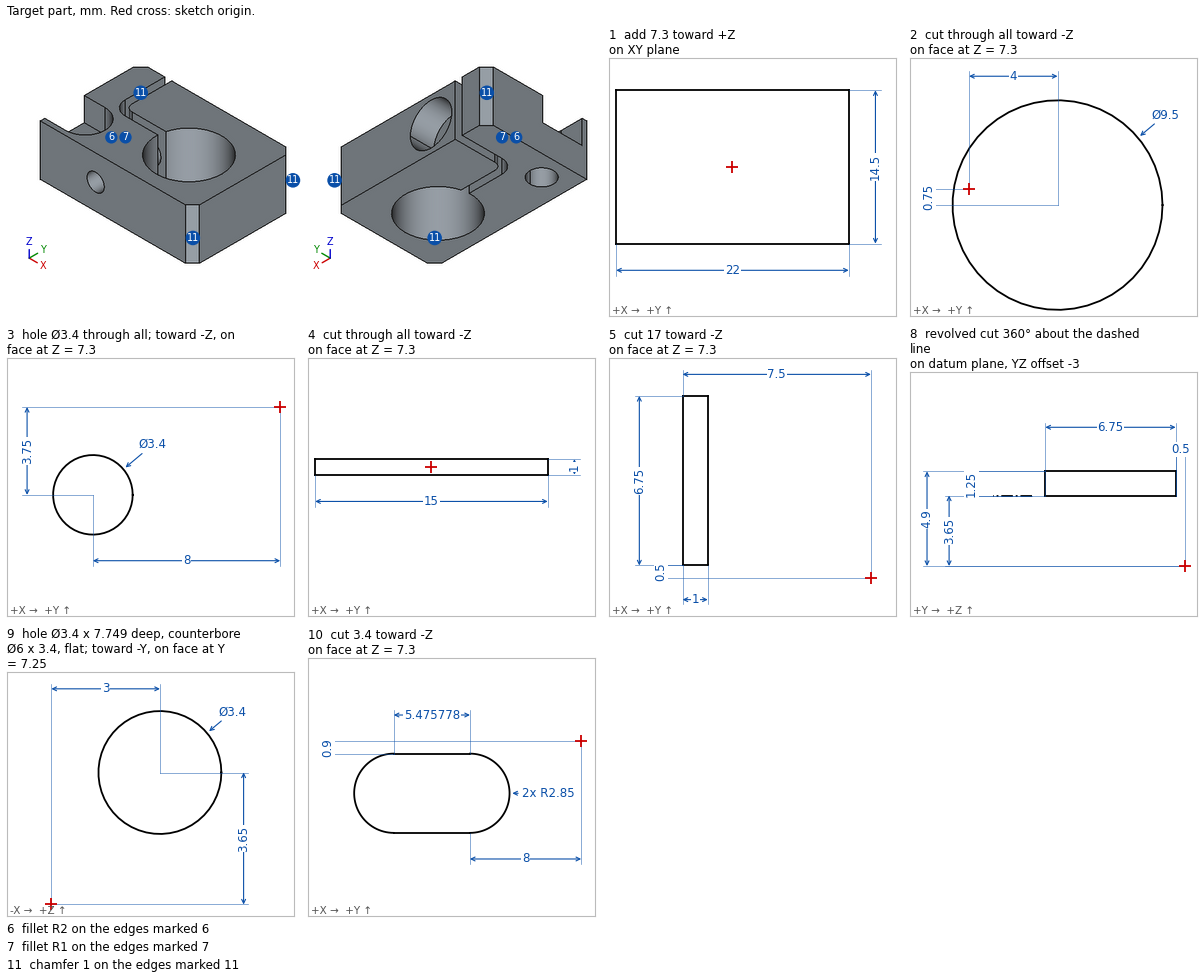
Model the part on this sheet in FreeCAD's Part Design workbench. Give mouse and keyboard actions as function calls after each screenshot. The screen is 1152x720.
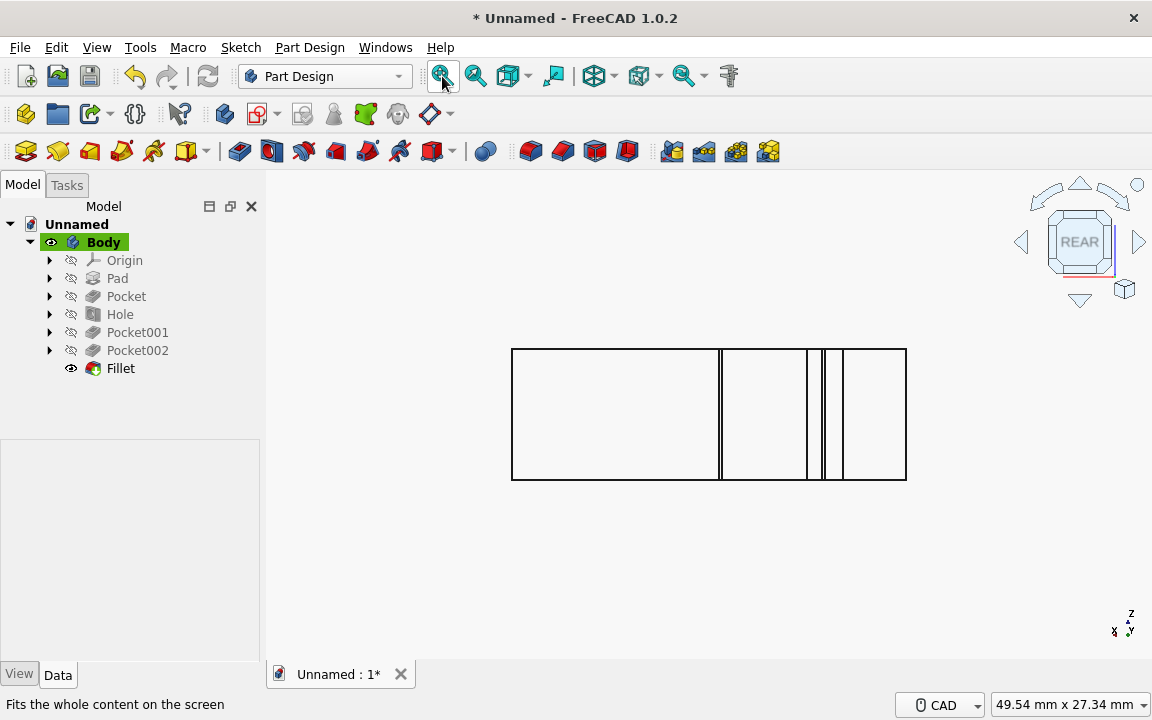
key(6)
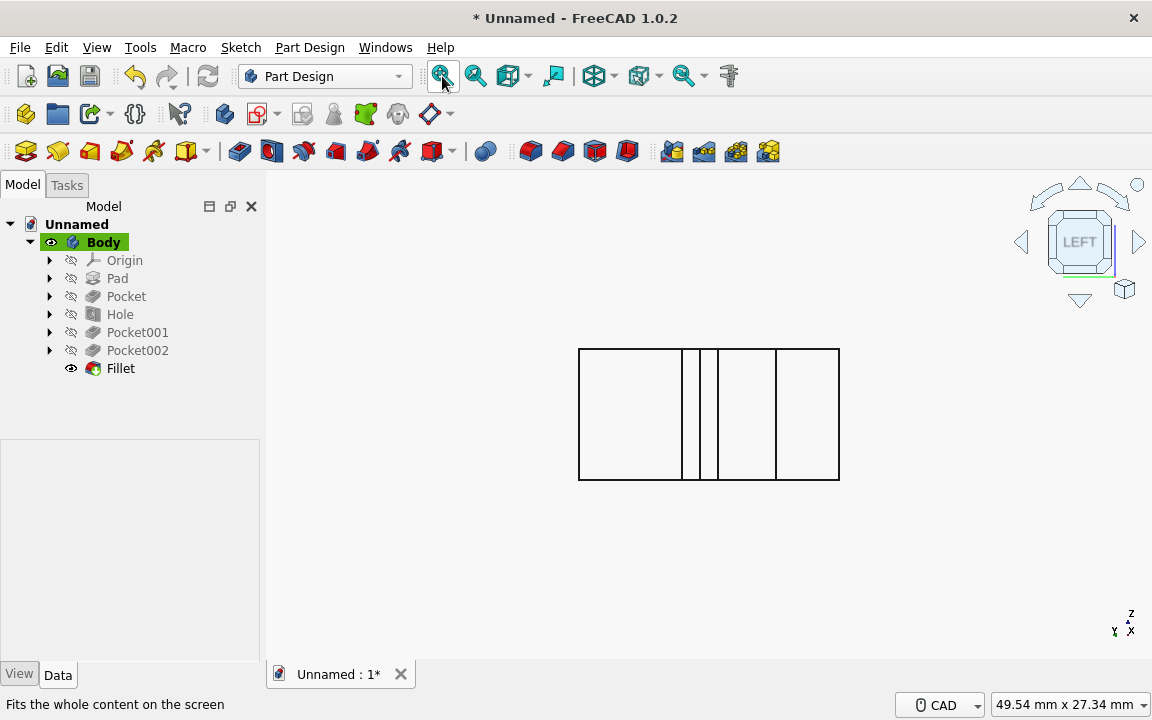
click(444, 76)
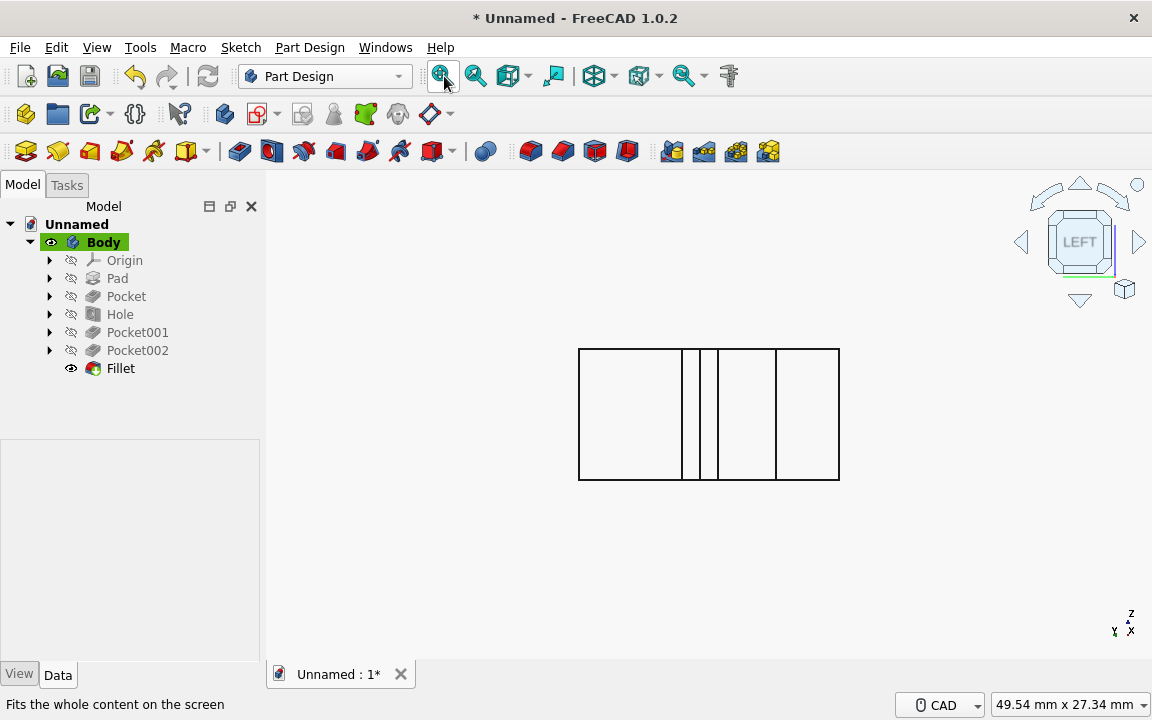
click(700, 413)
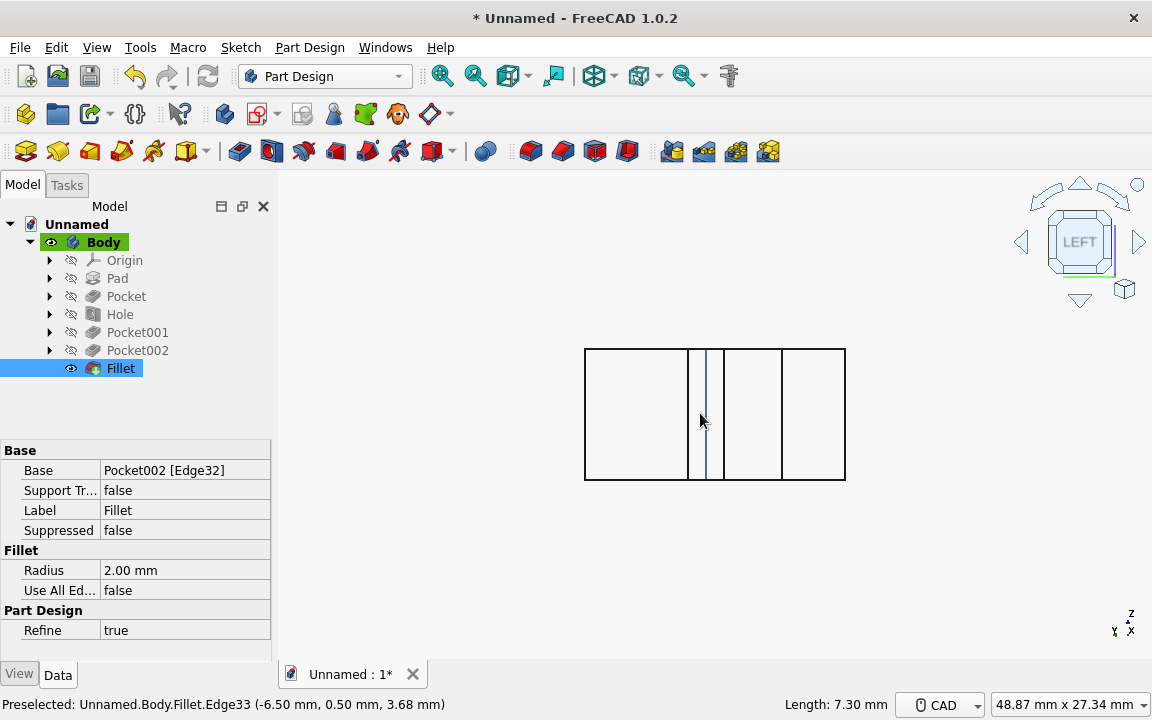
key(v)
key(1)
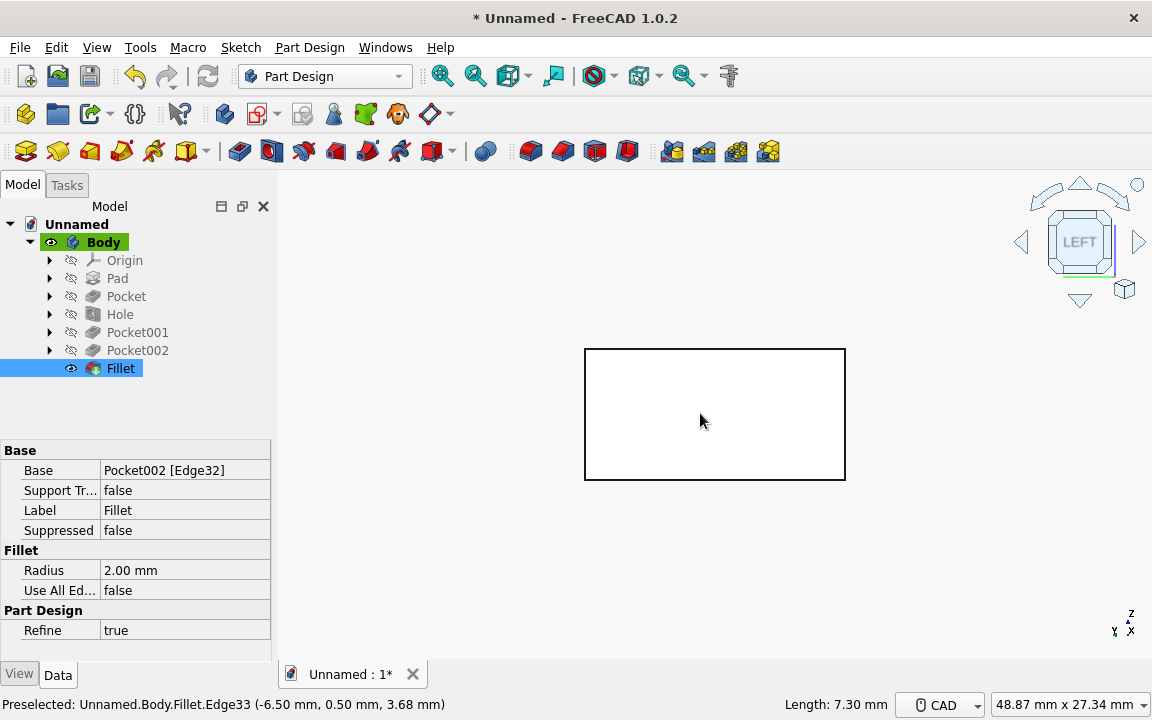
click(532, 152)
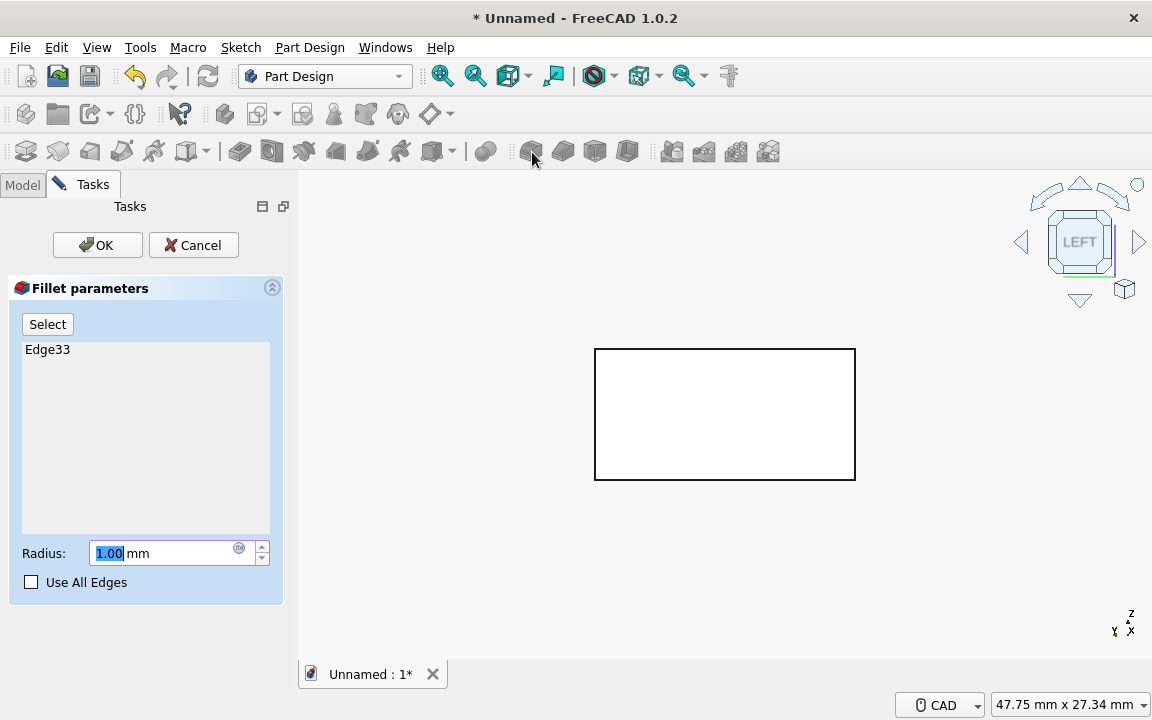
text(1)
key(Tab)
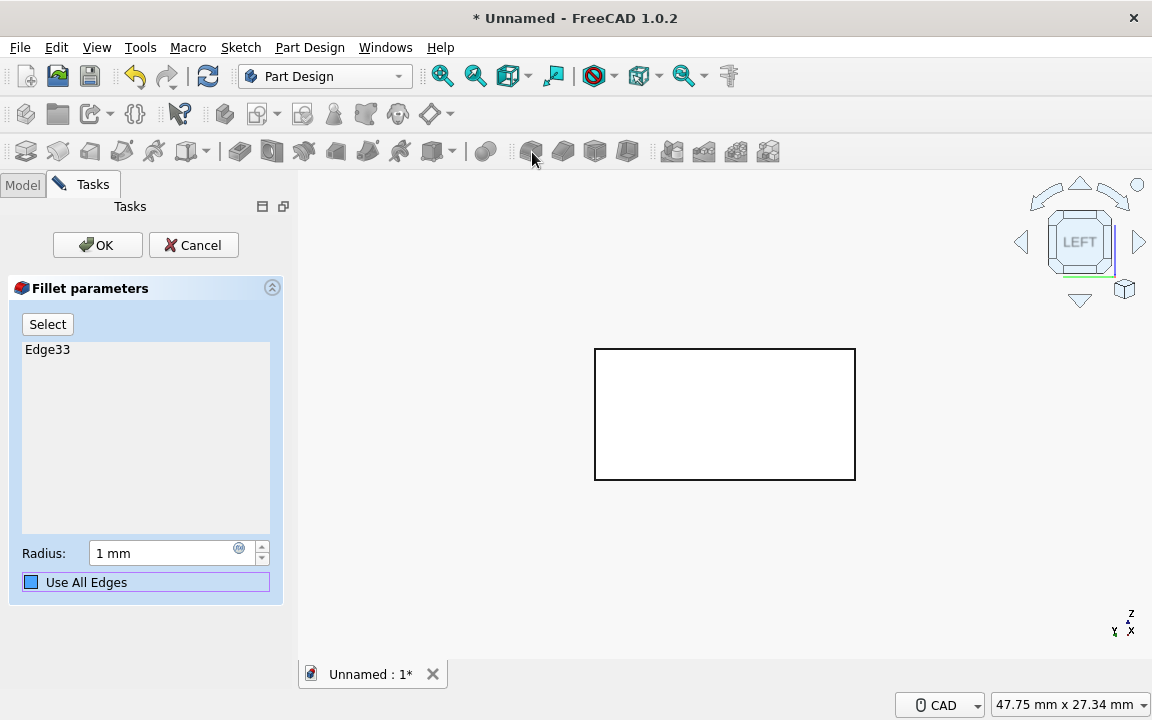
click(98, 245)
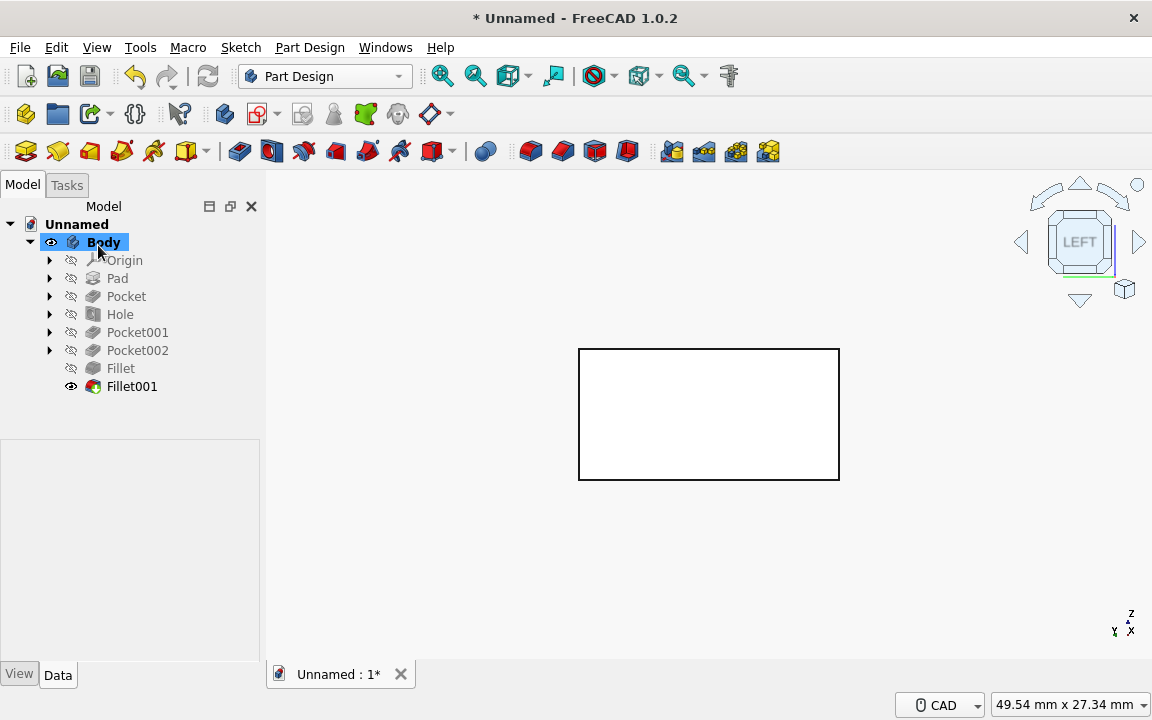
click(444, 76)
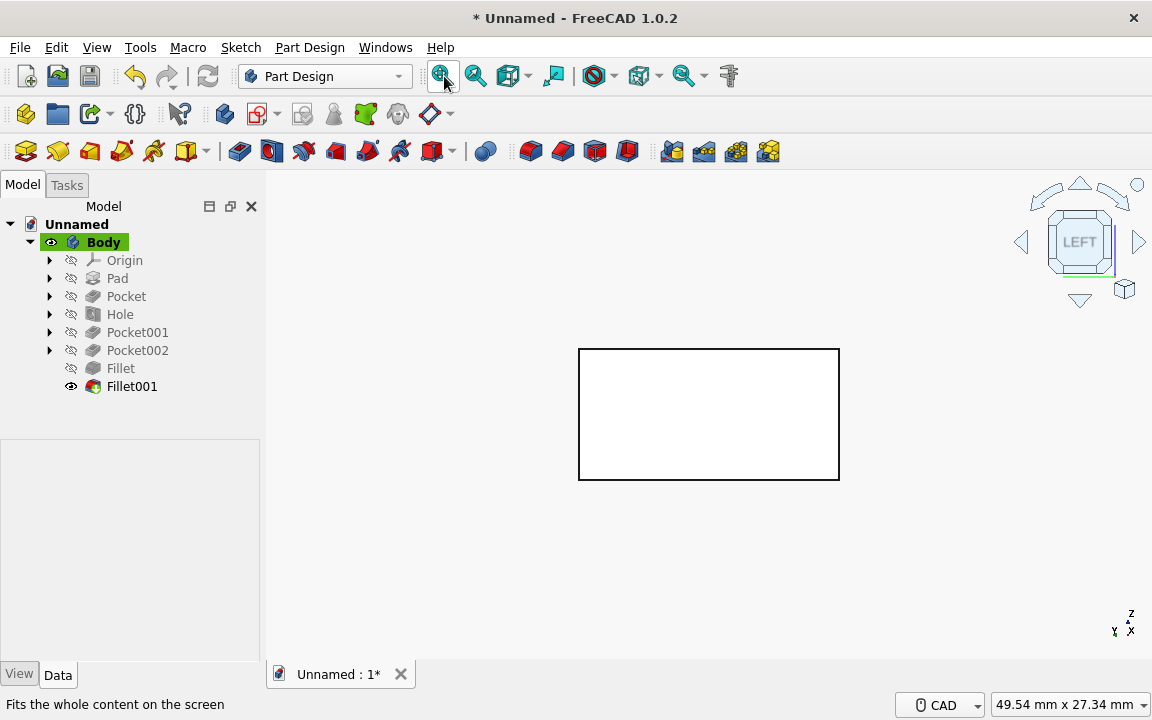
click(50, 260)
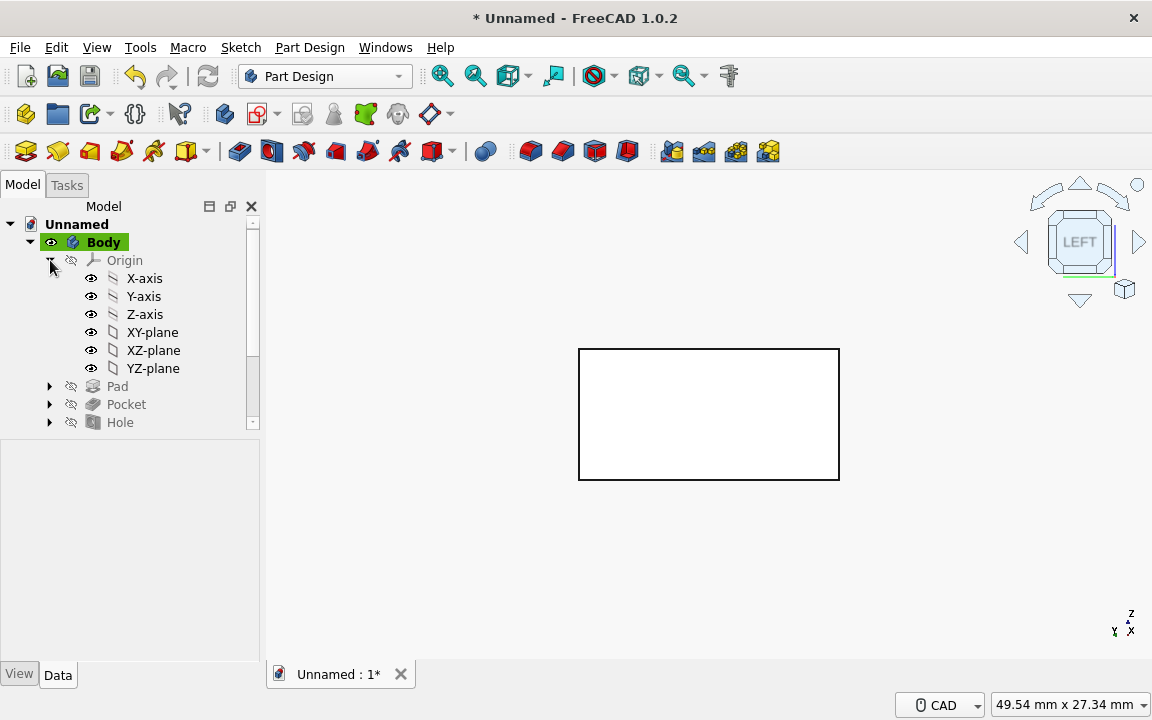
click(136, 368)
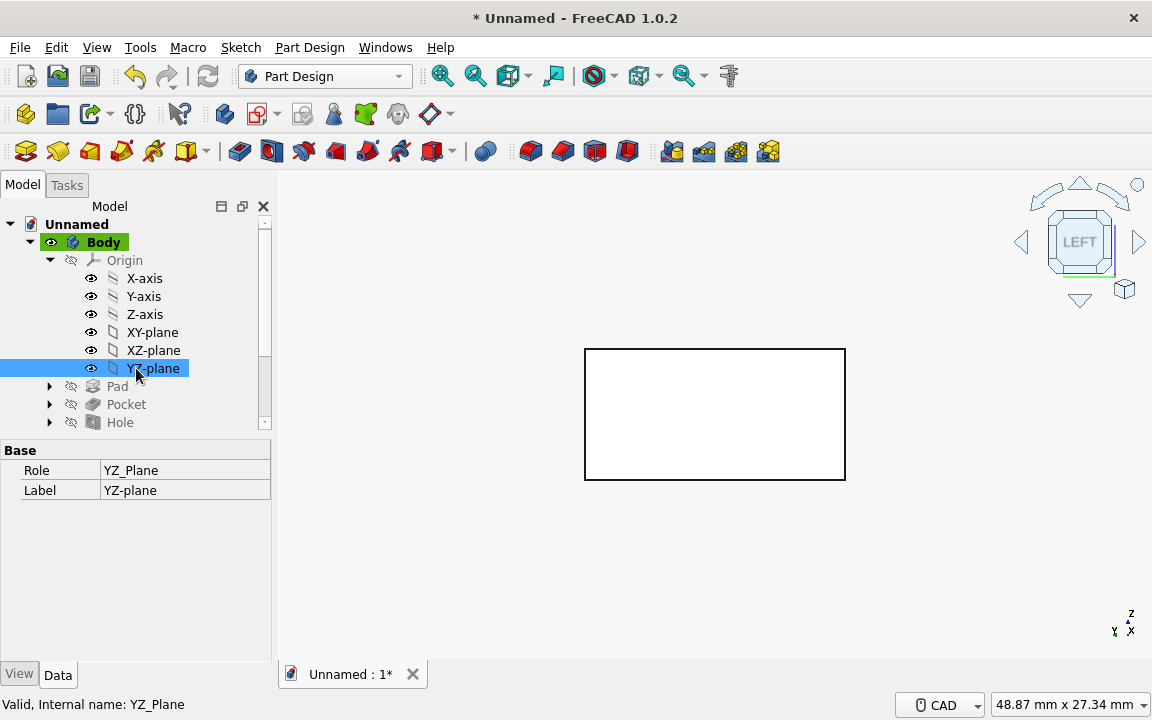
click(430, 114)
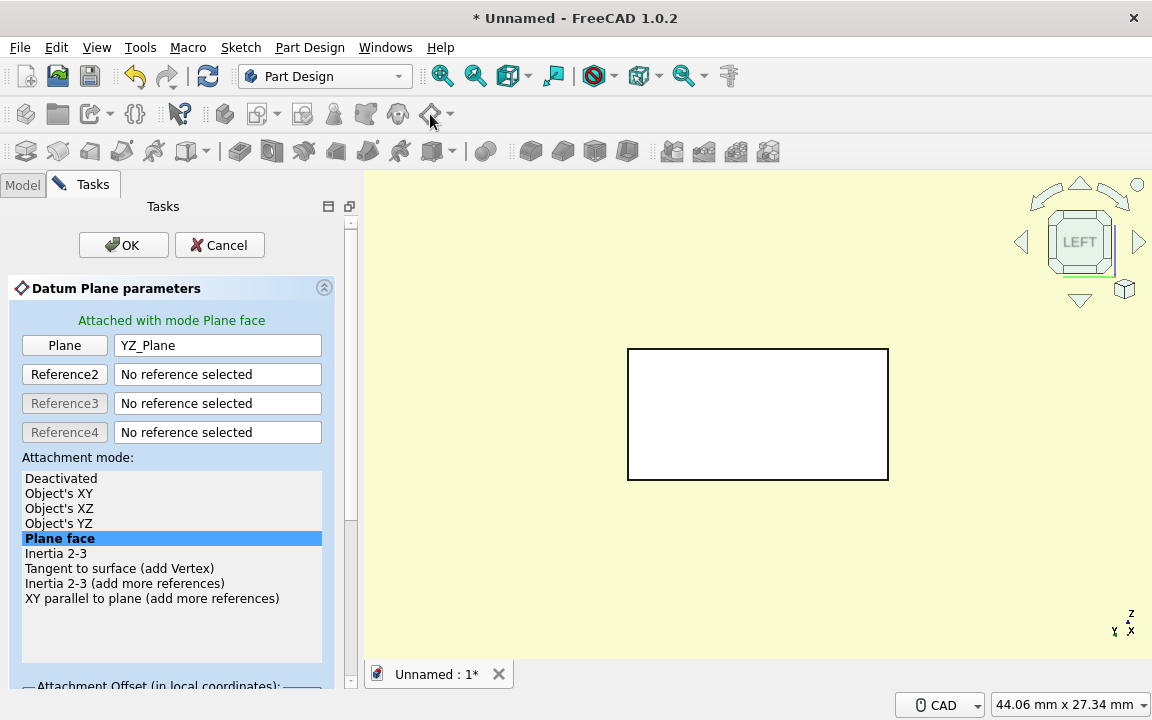
scroll(351, 452, down, 3)